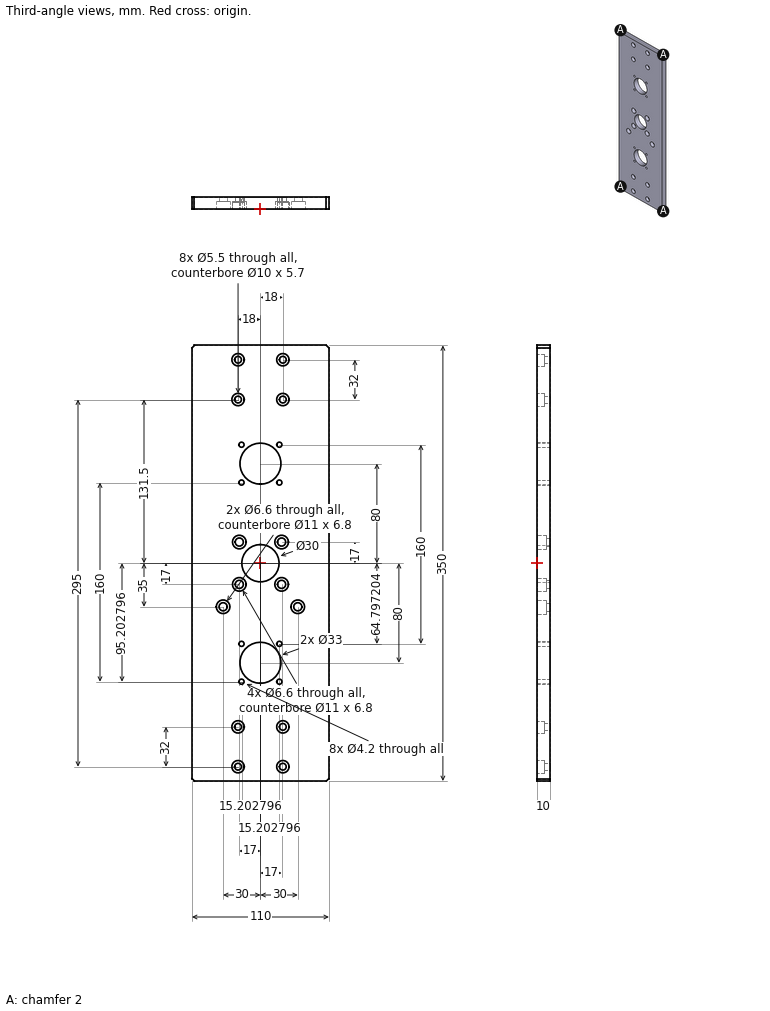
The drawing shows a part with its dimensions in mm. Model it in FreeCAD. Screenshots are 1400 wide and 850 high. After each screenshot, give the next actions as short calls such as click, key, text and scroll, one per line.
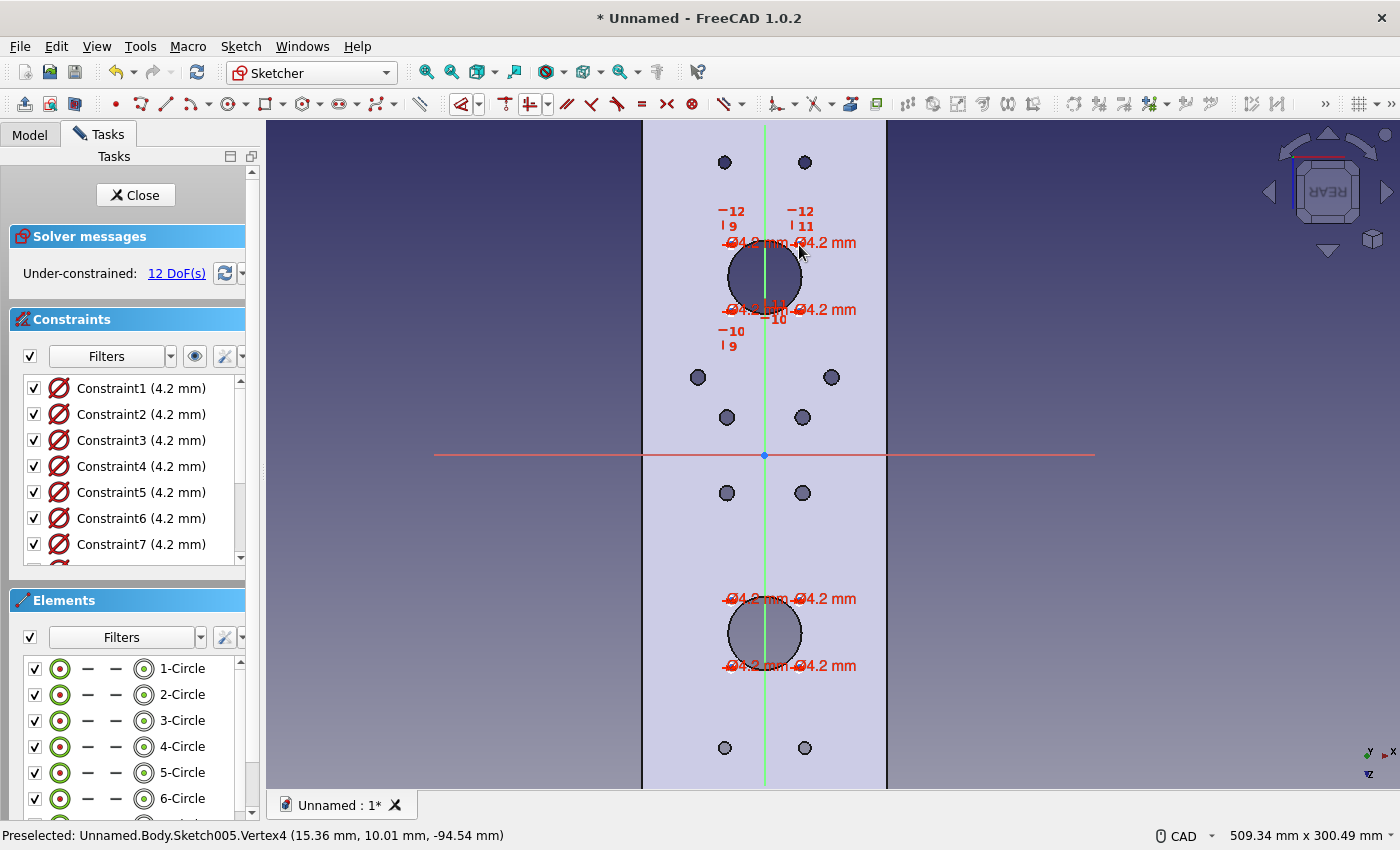
click(731, 312)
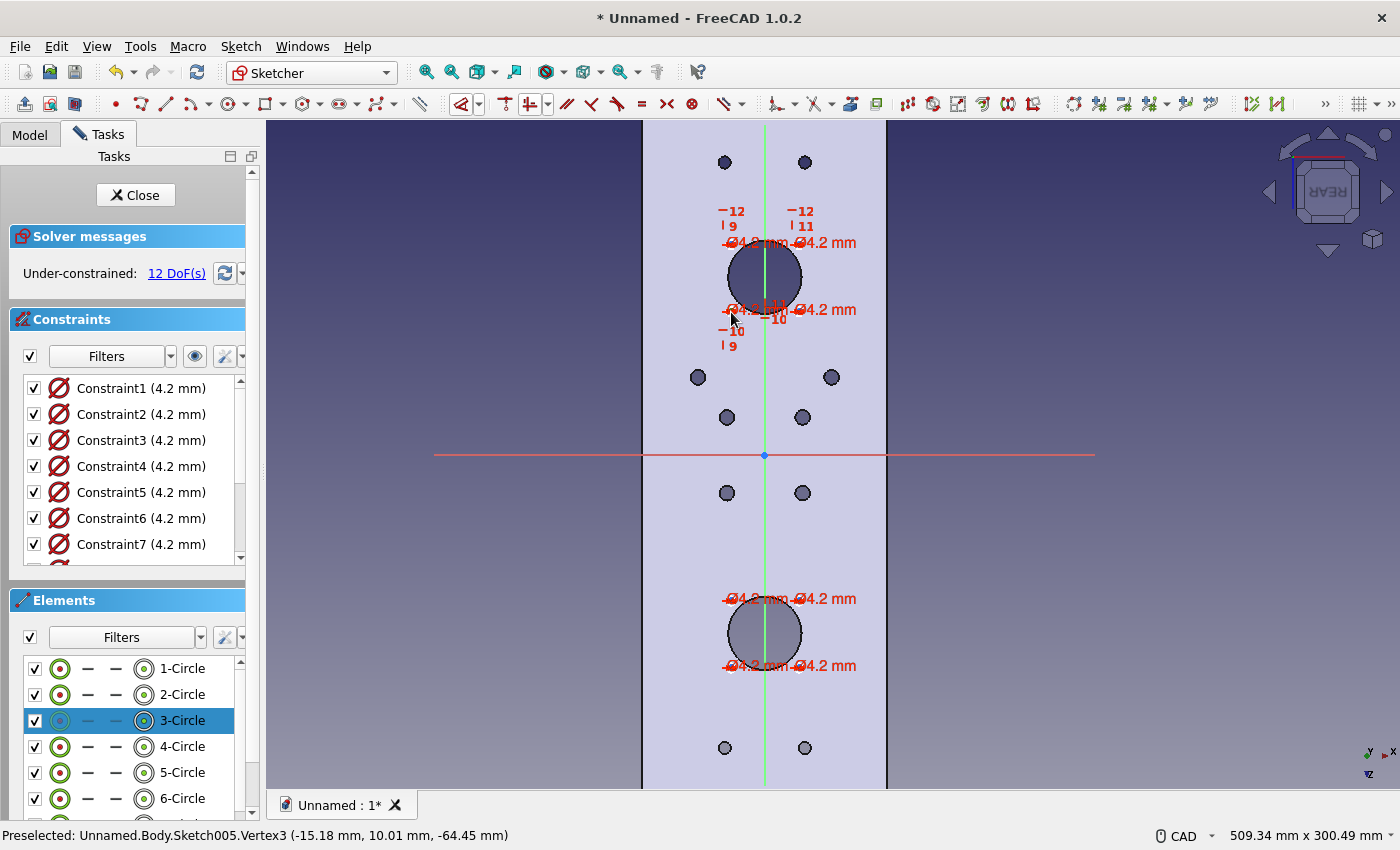
click(731, 601)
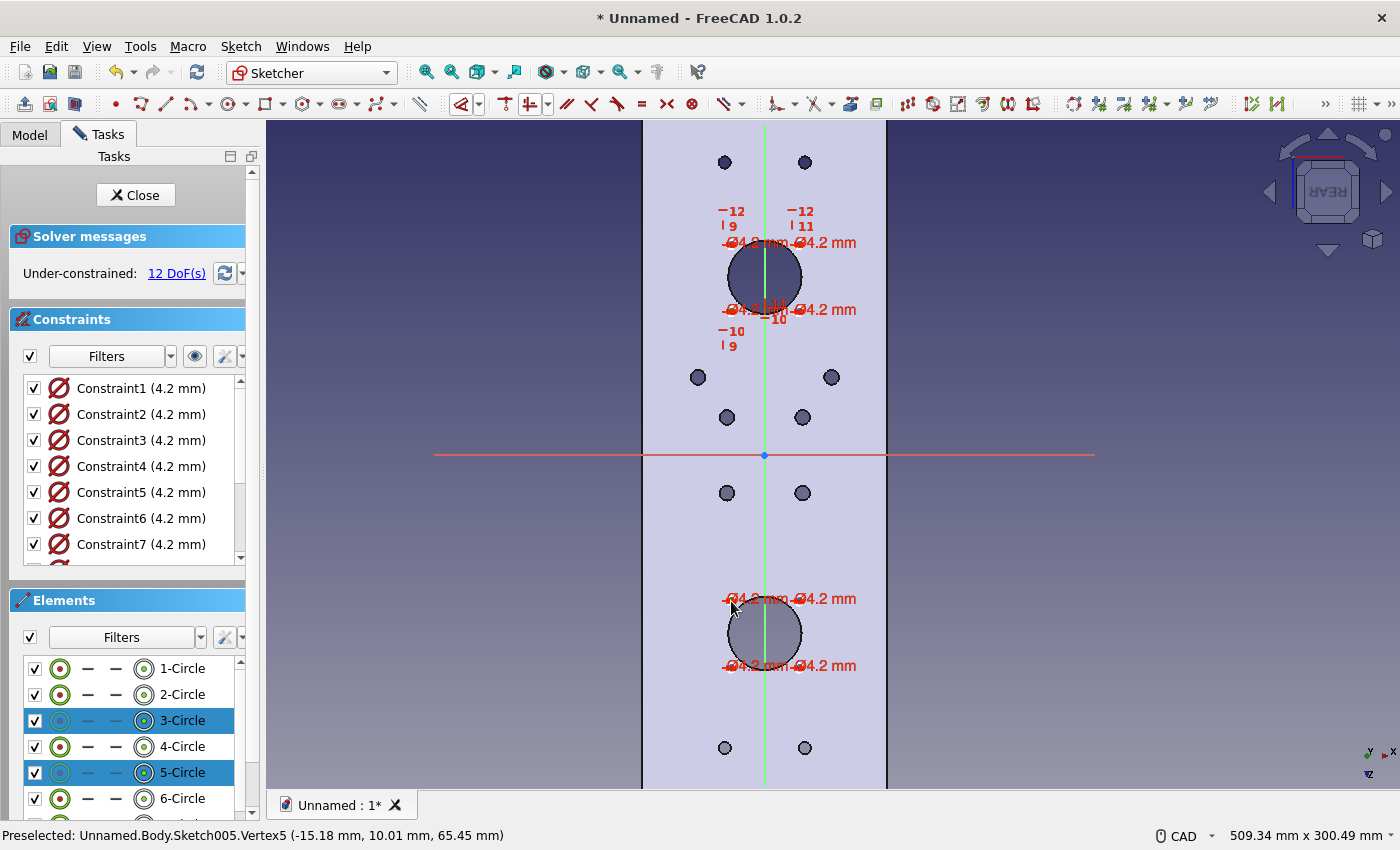
key(v)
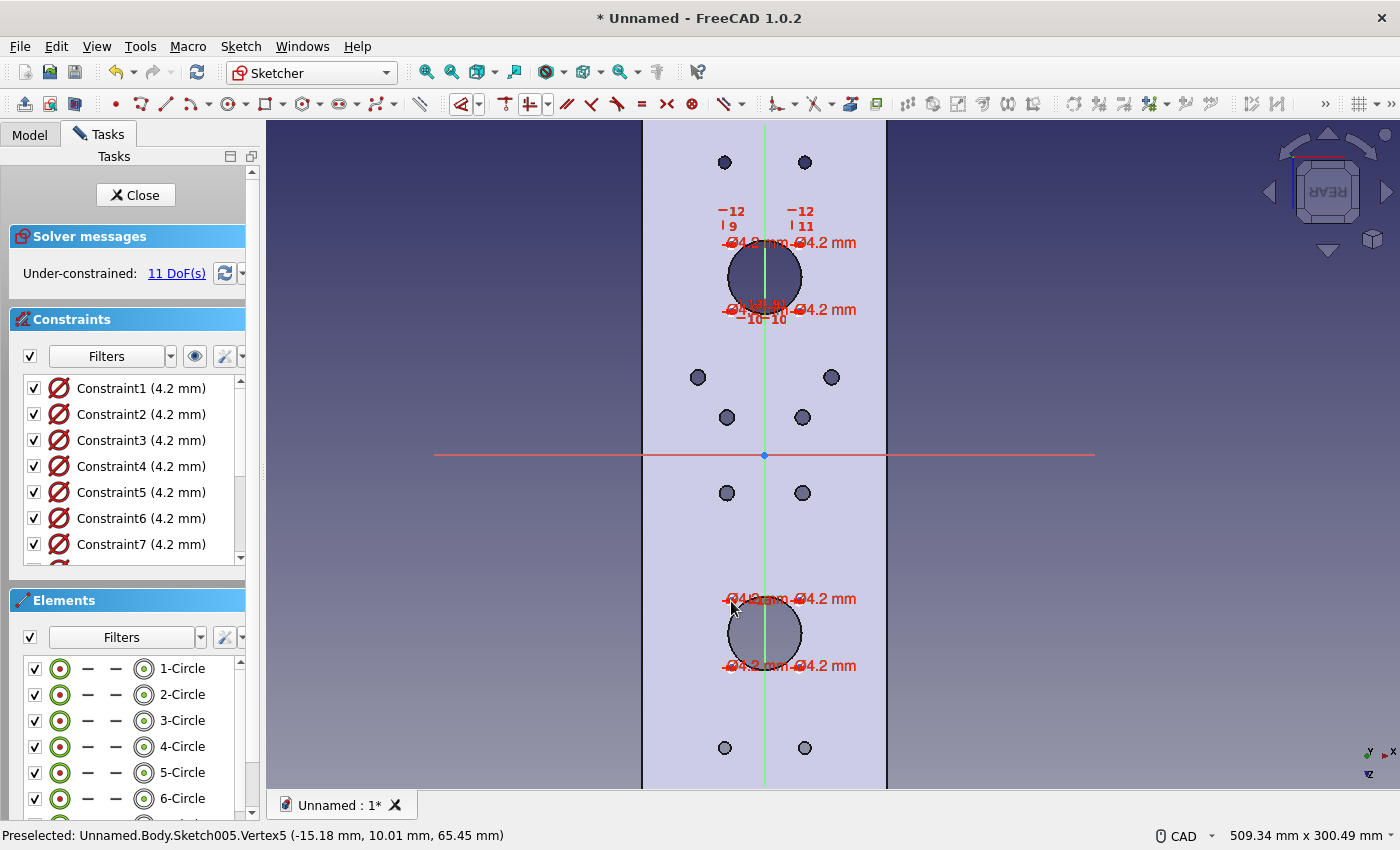
click(799, 312)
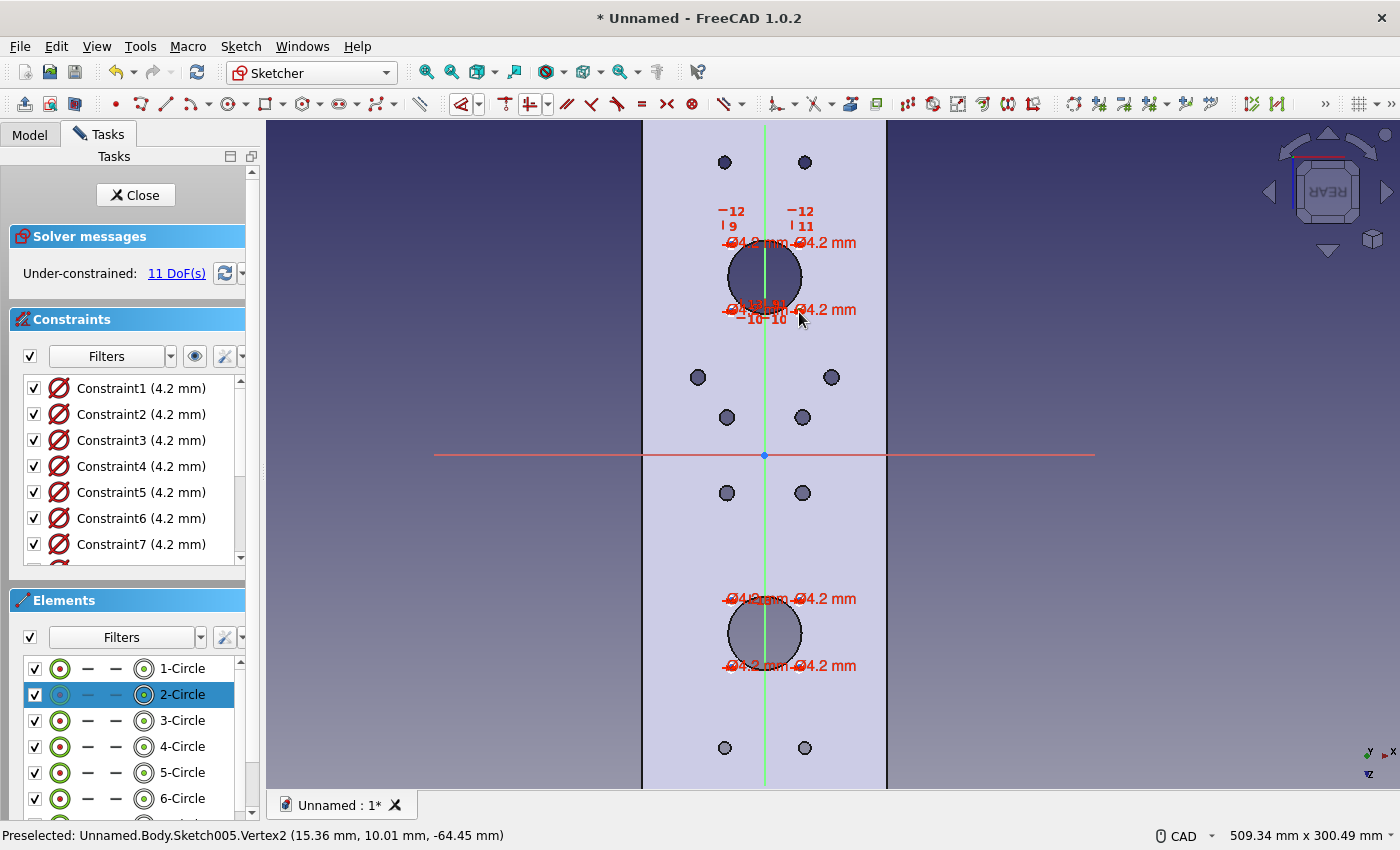
click(799, 668)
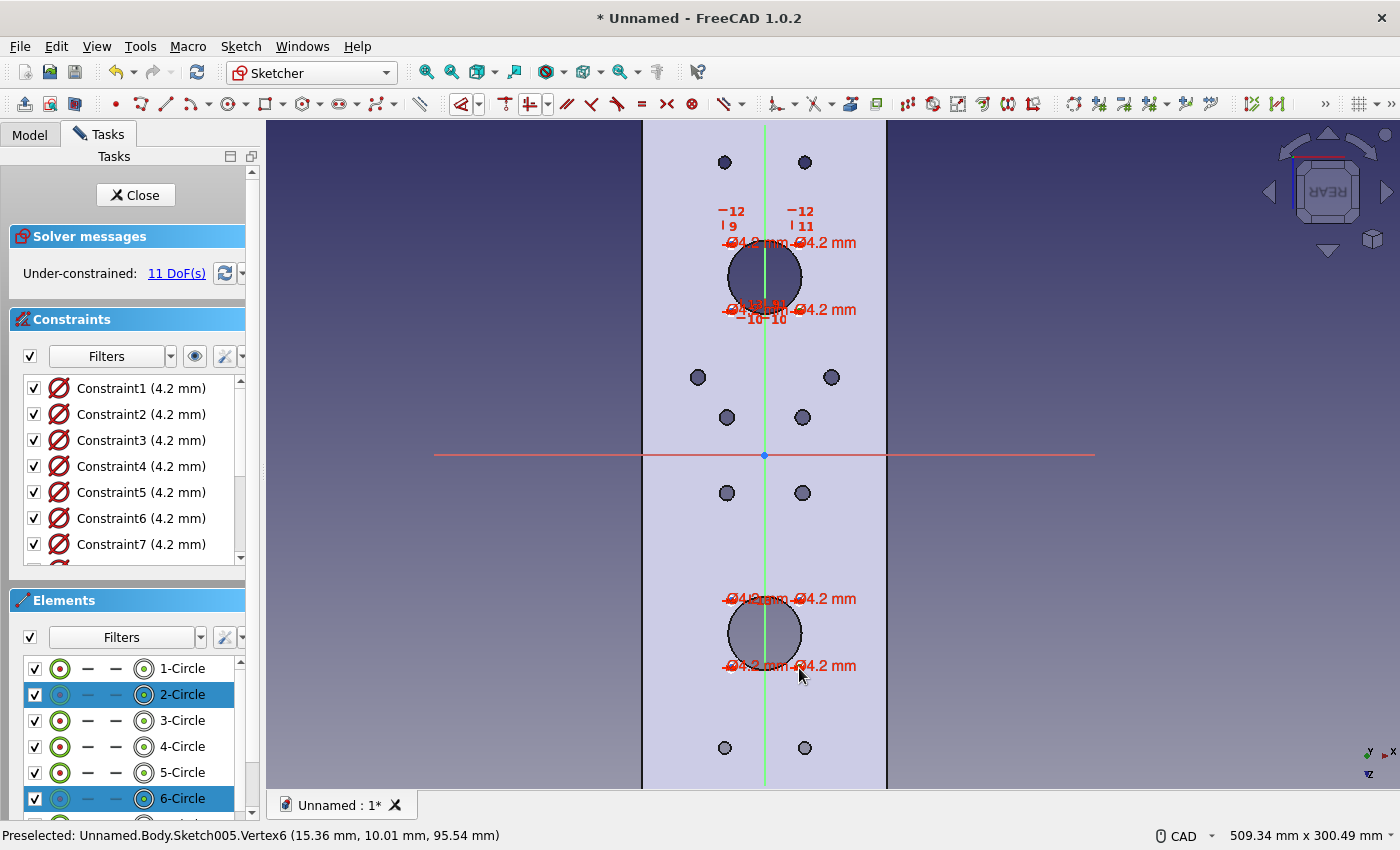
key(v)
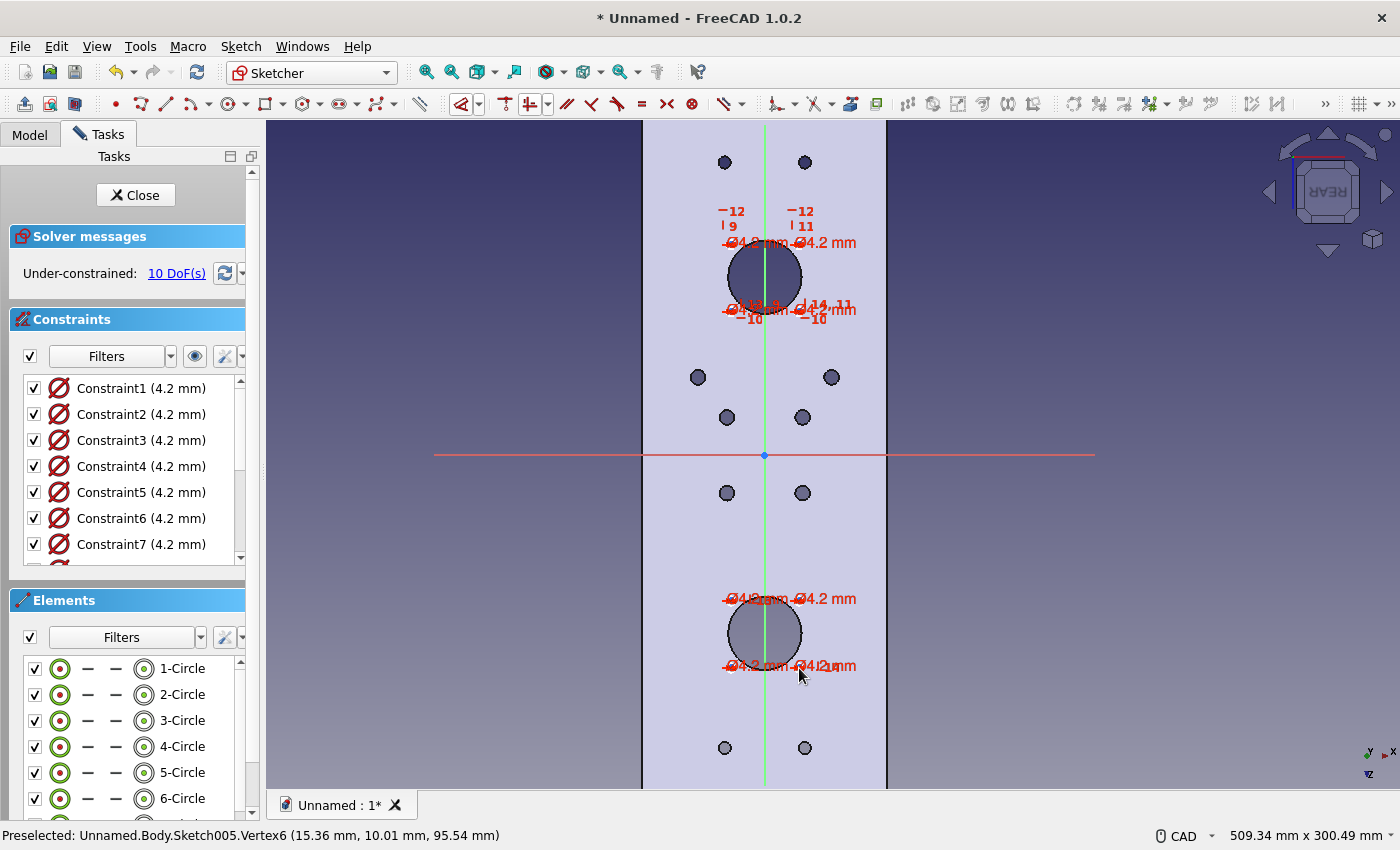
click(799, 668)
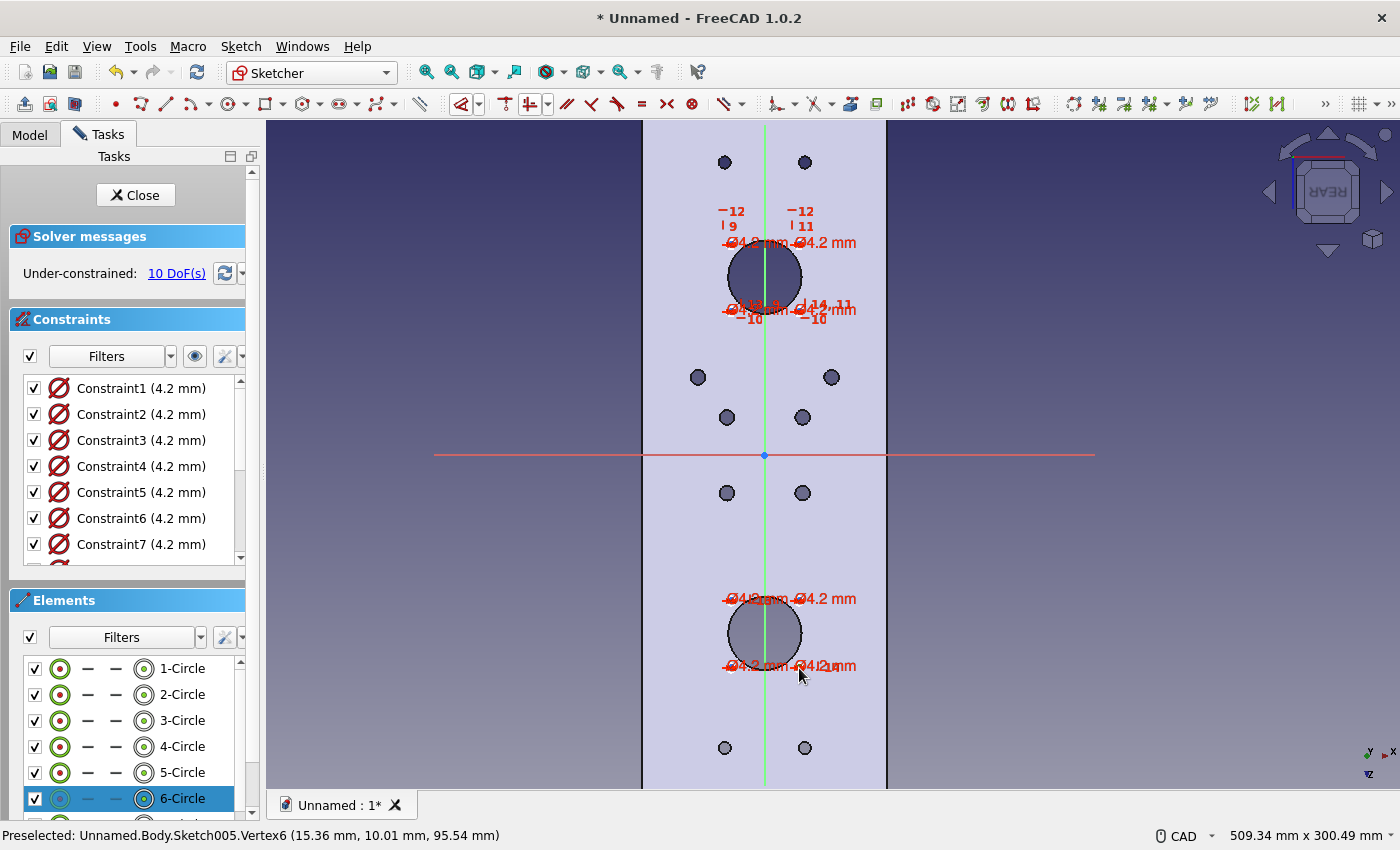
click(799, 601)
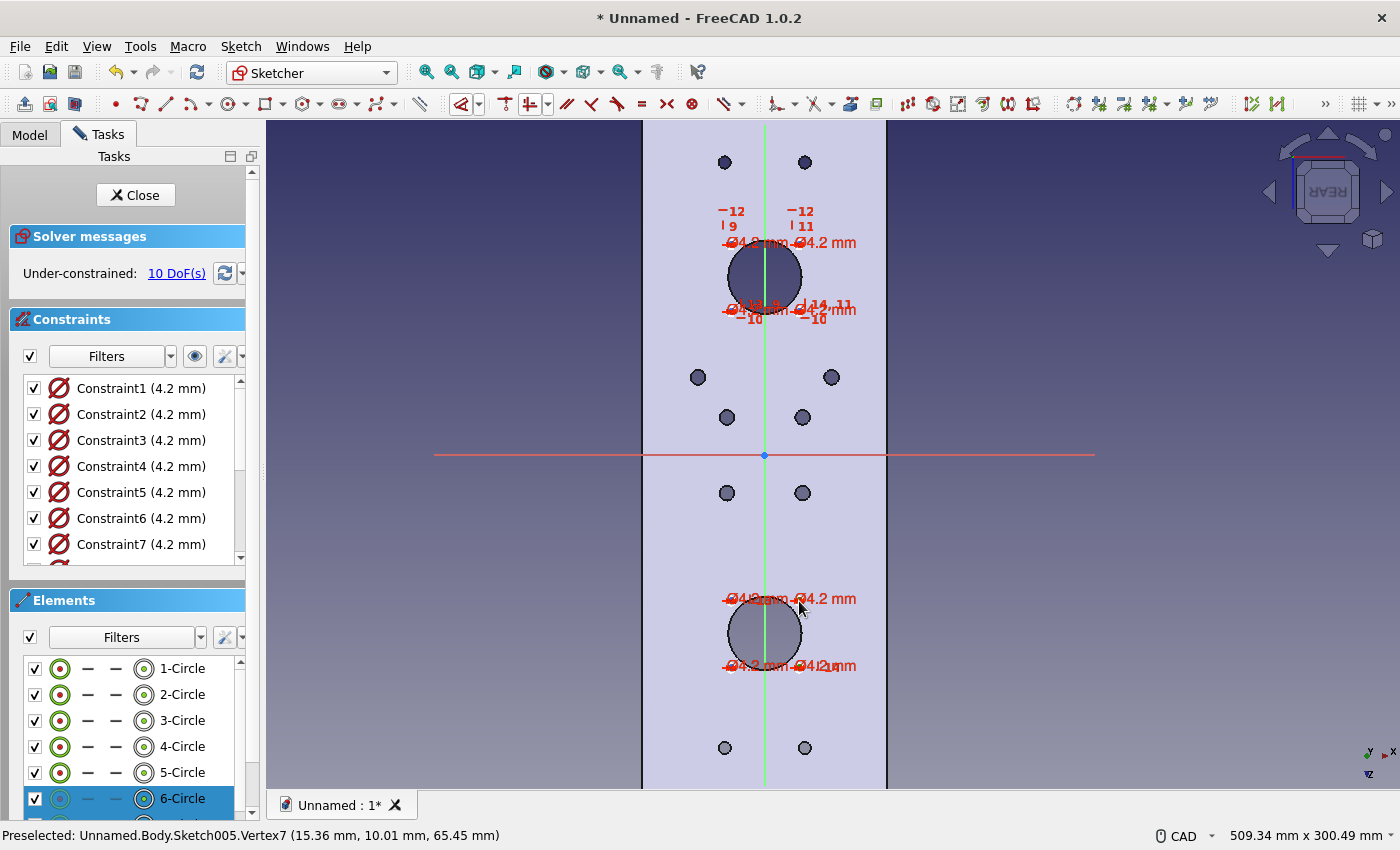
click(548, 104)